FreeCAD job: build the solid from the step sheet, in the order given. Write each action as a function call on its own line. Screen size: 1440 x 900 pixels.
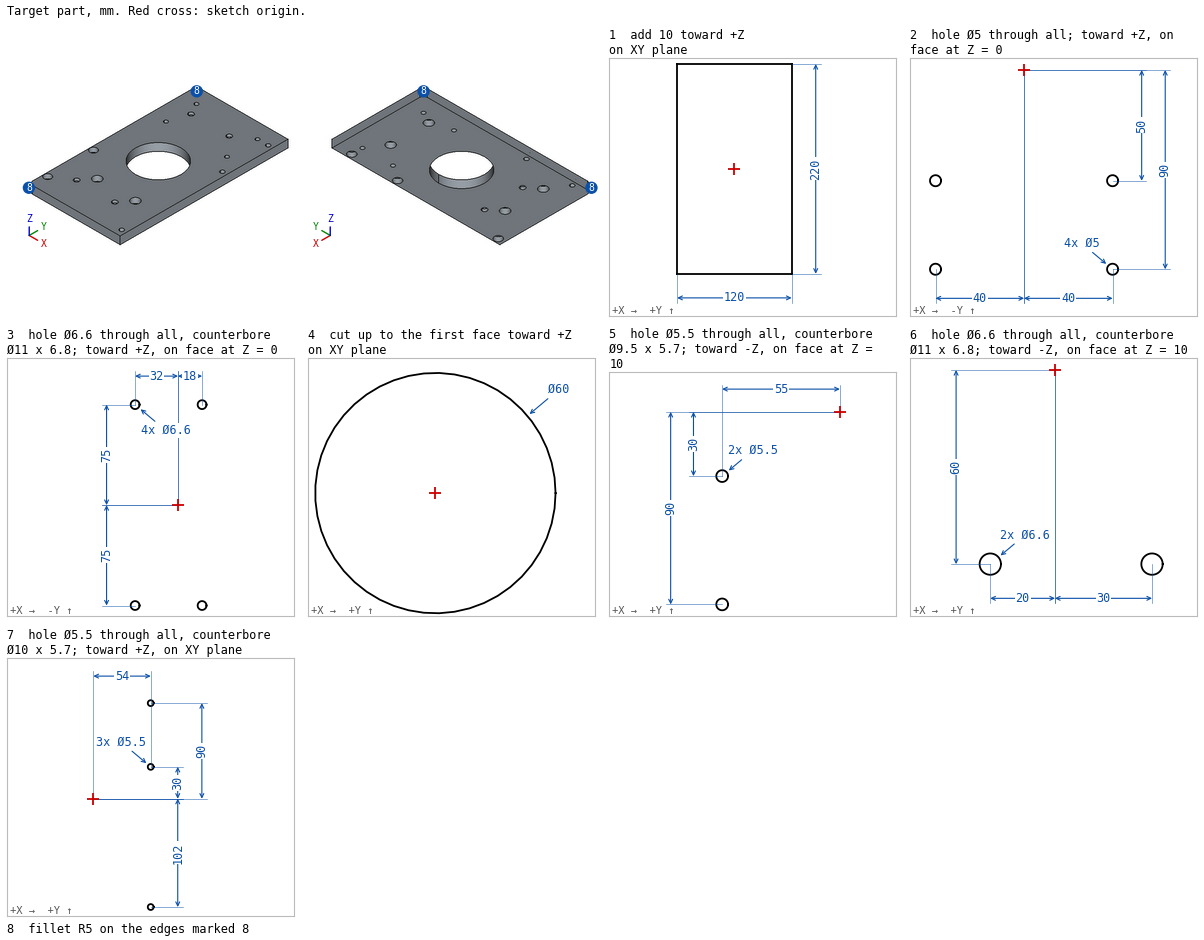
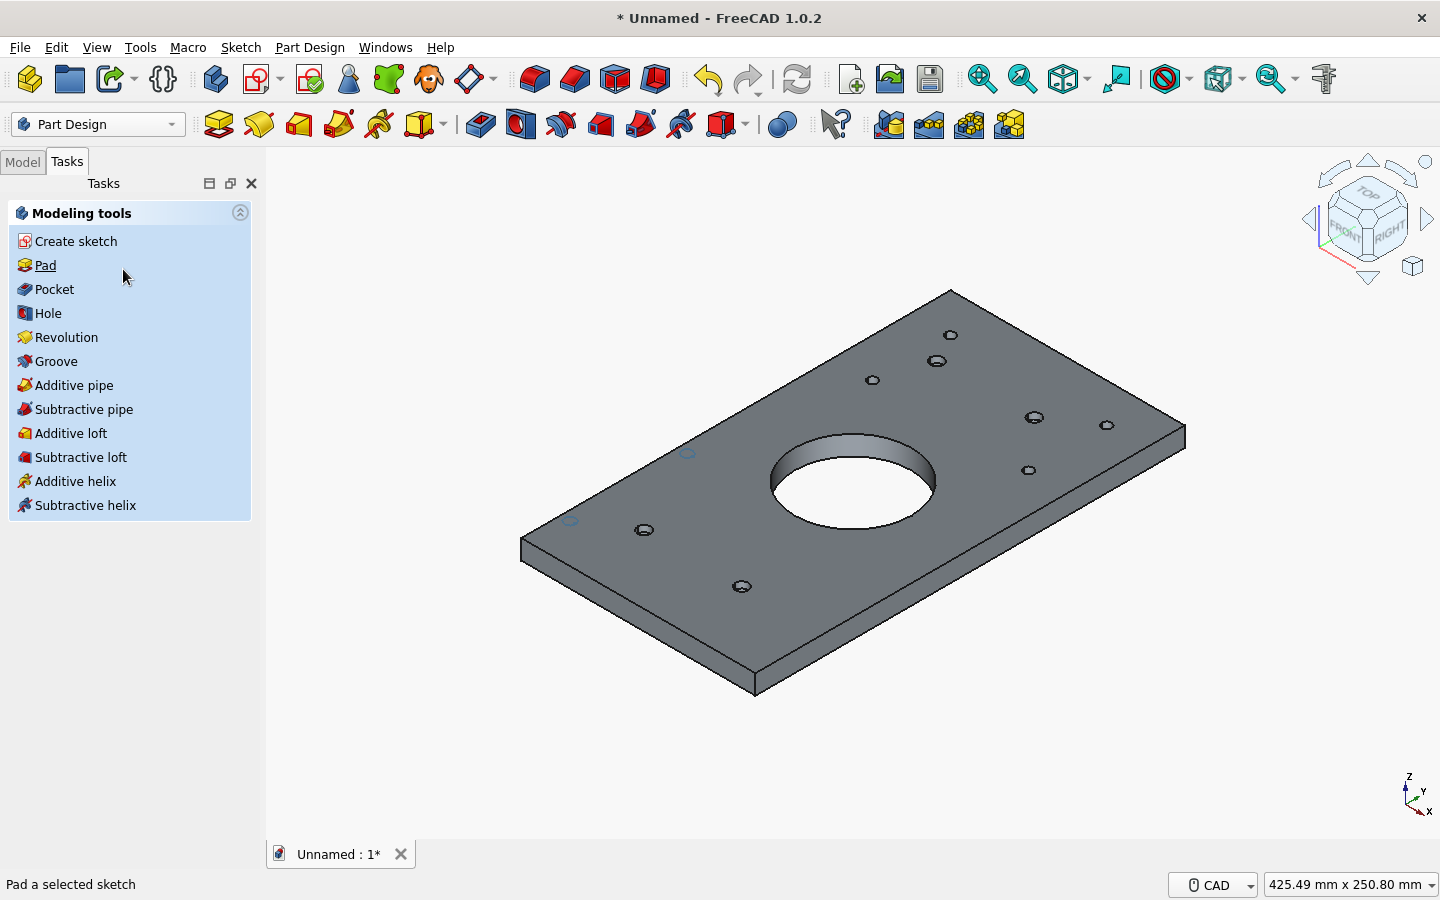
click(522, 124)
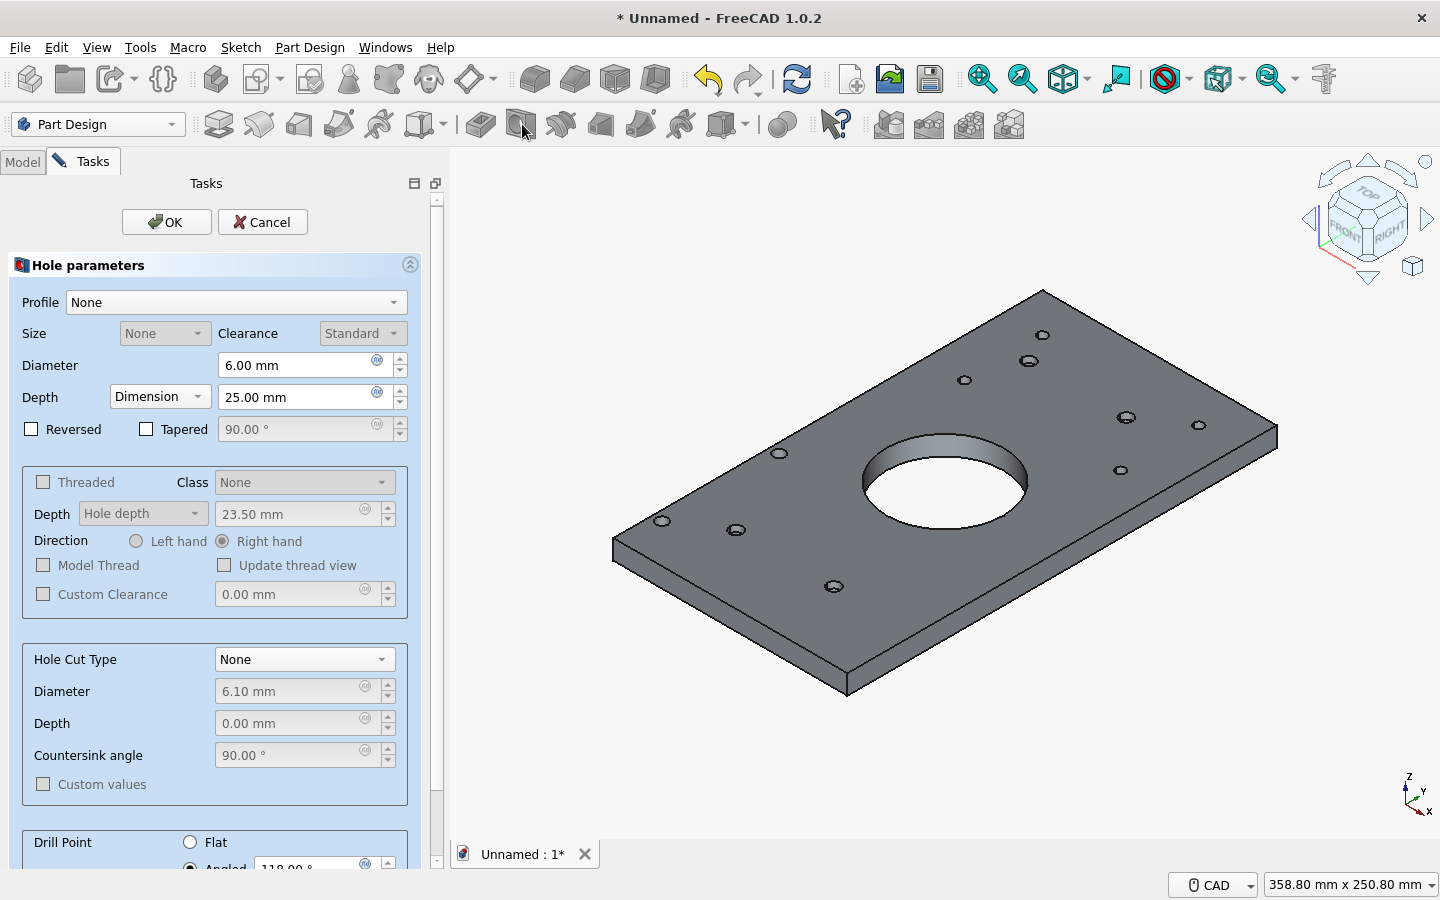
triple_click(305, 365)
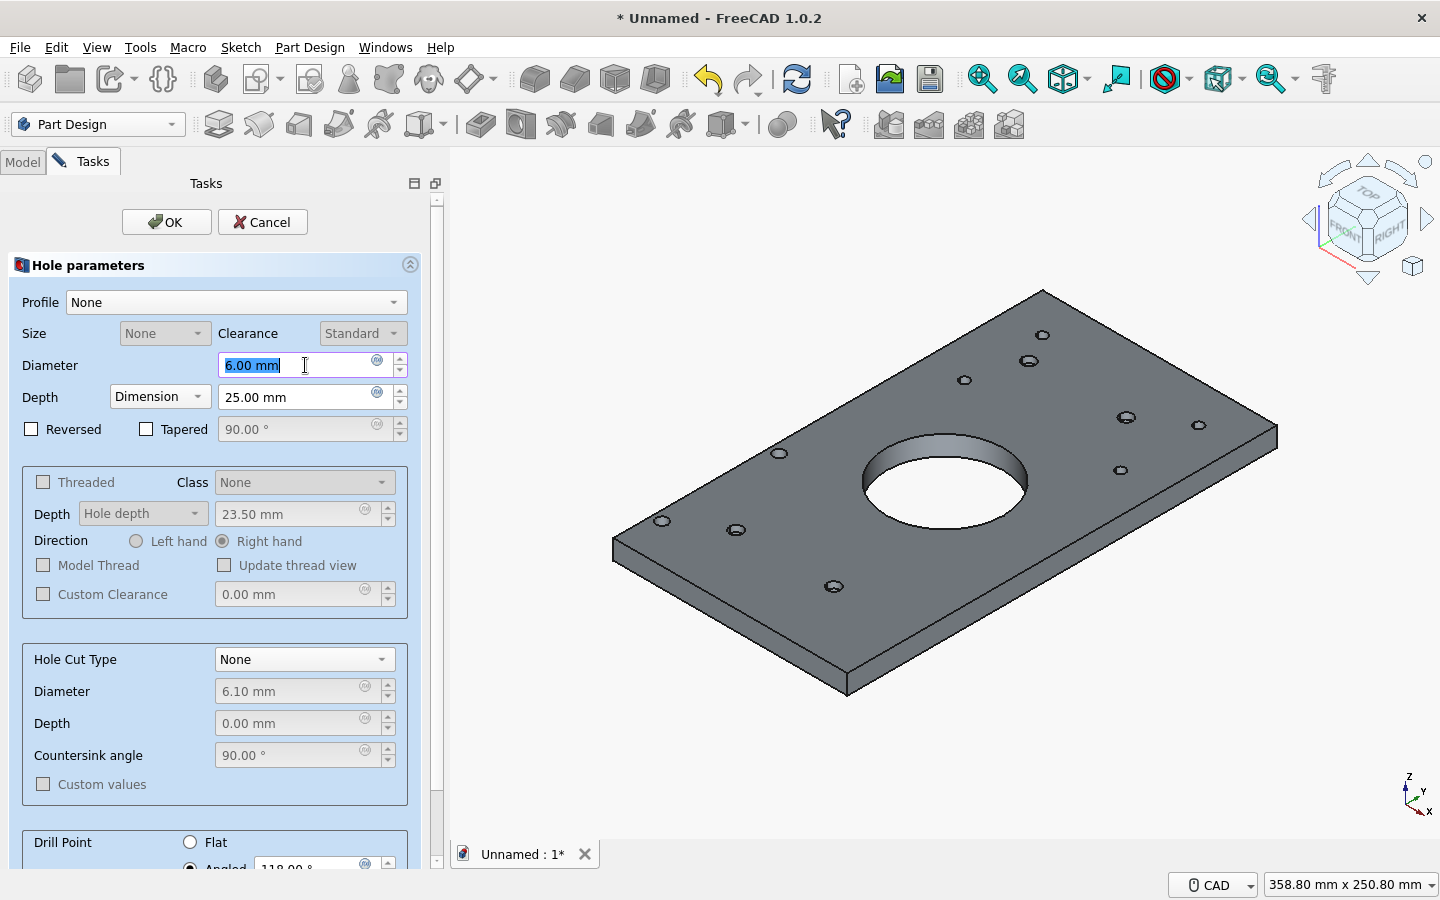
text(5.5)
key(Tab)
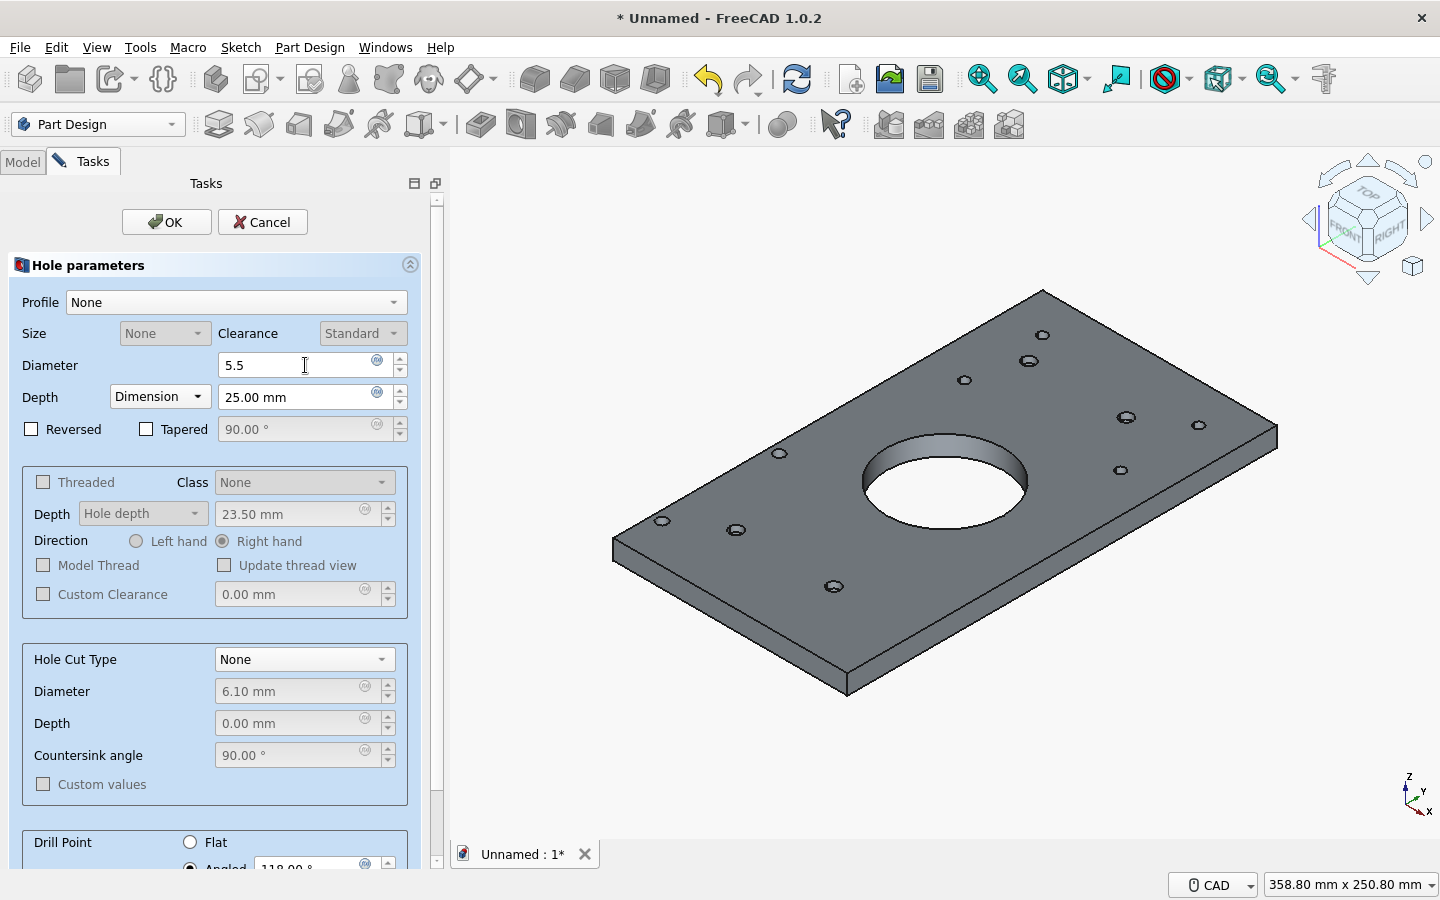
click(161, 396)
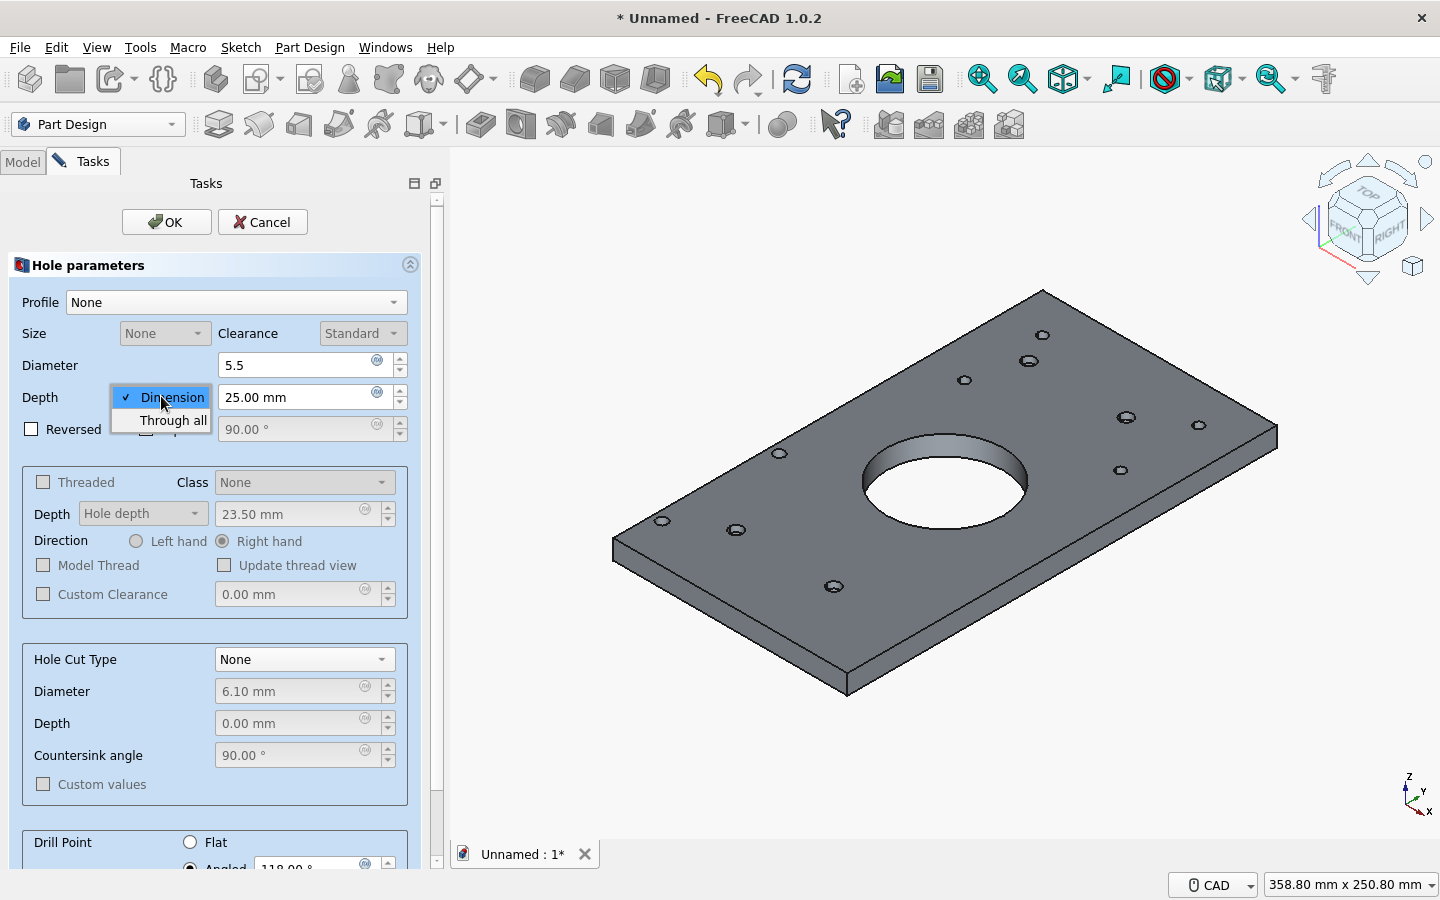
click(160, 420)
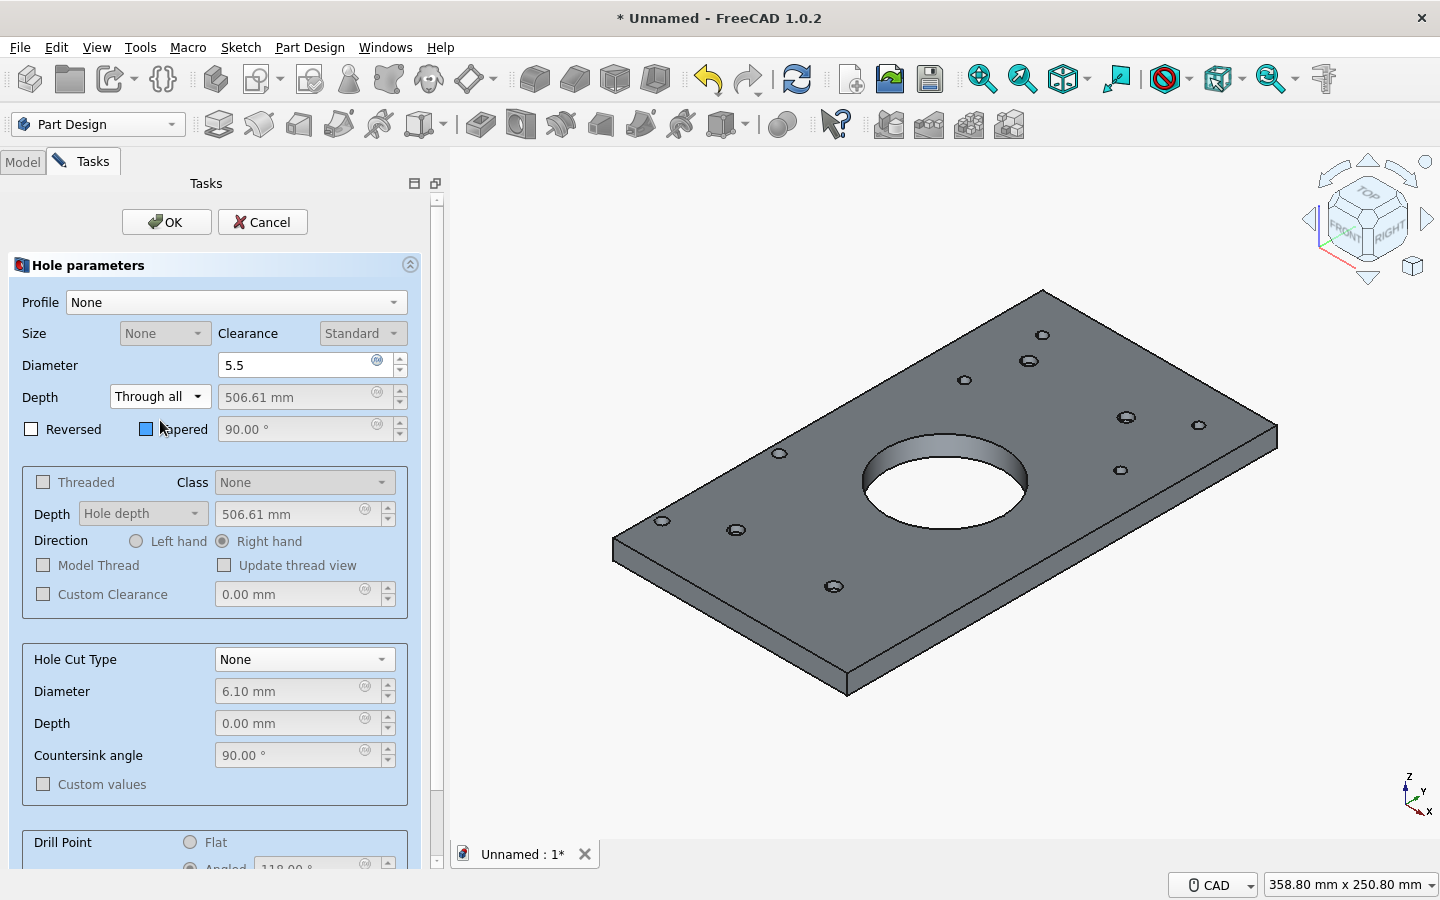
click(306, 660)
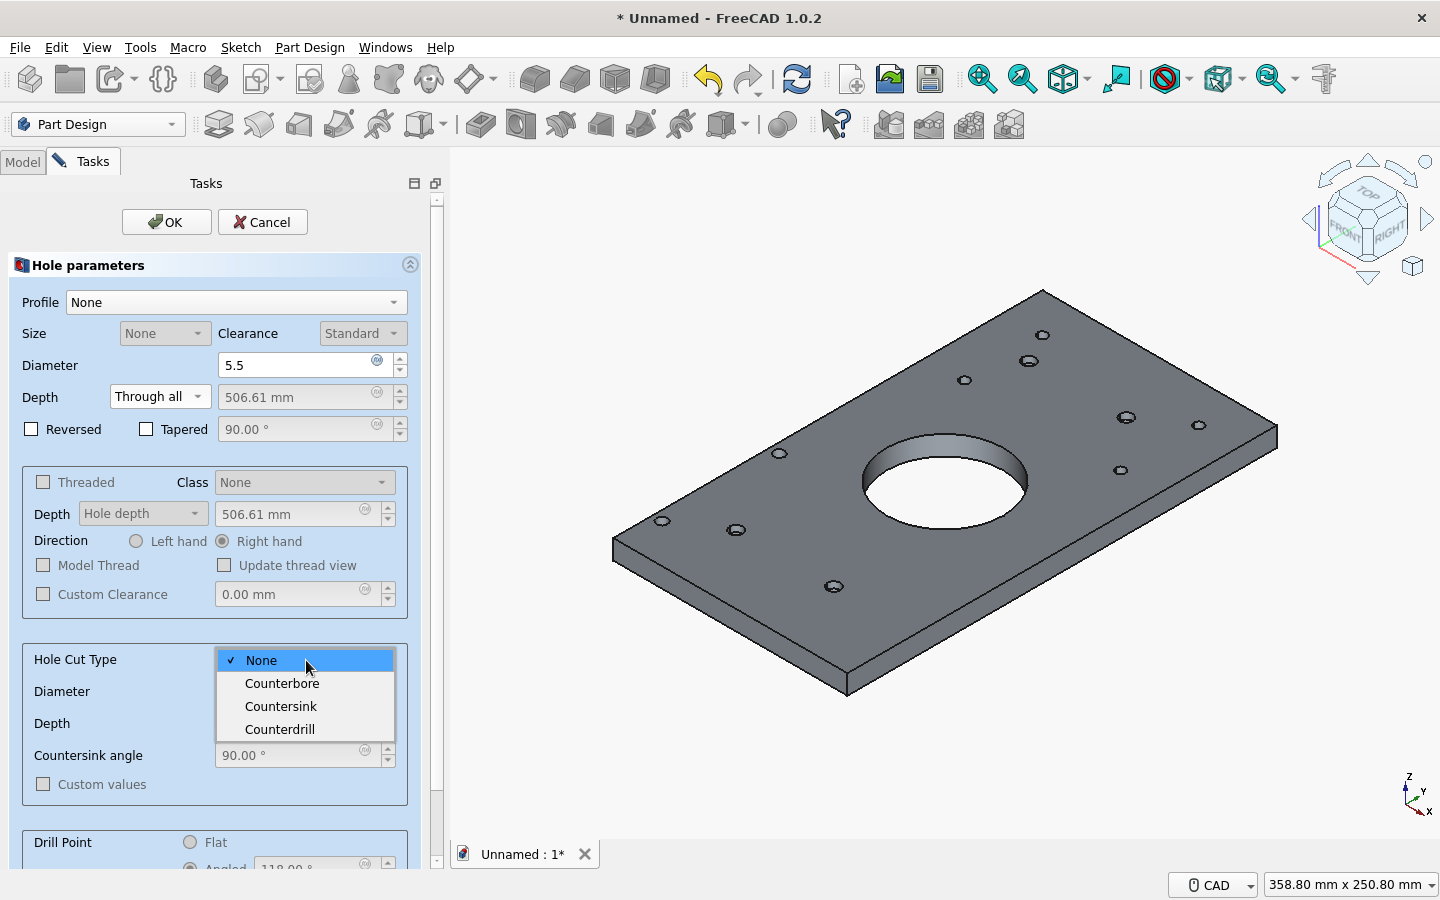
click(304, 684)